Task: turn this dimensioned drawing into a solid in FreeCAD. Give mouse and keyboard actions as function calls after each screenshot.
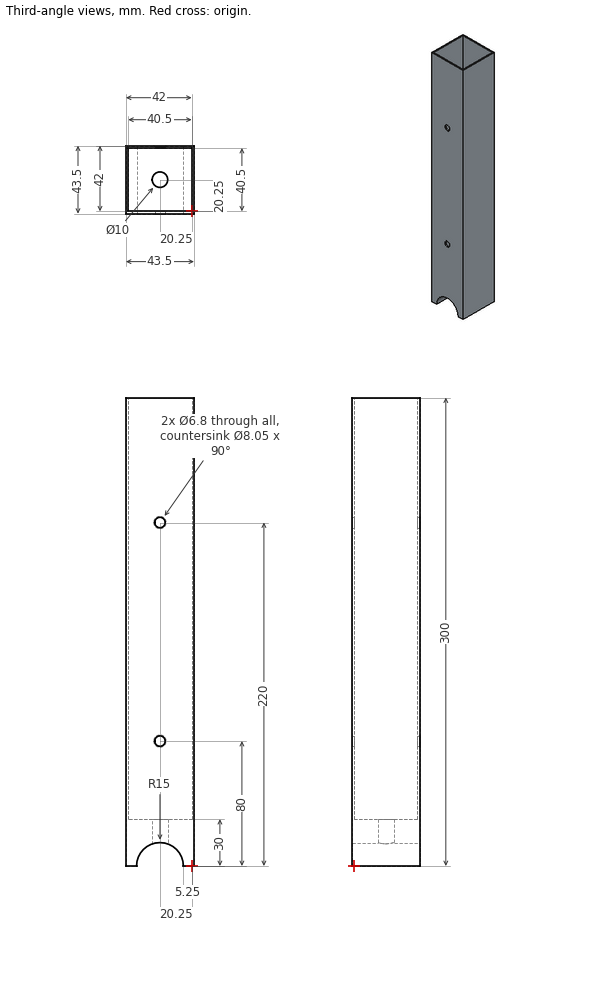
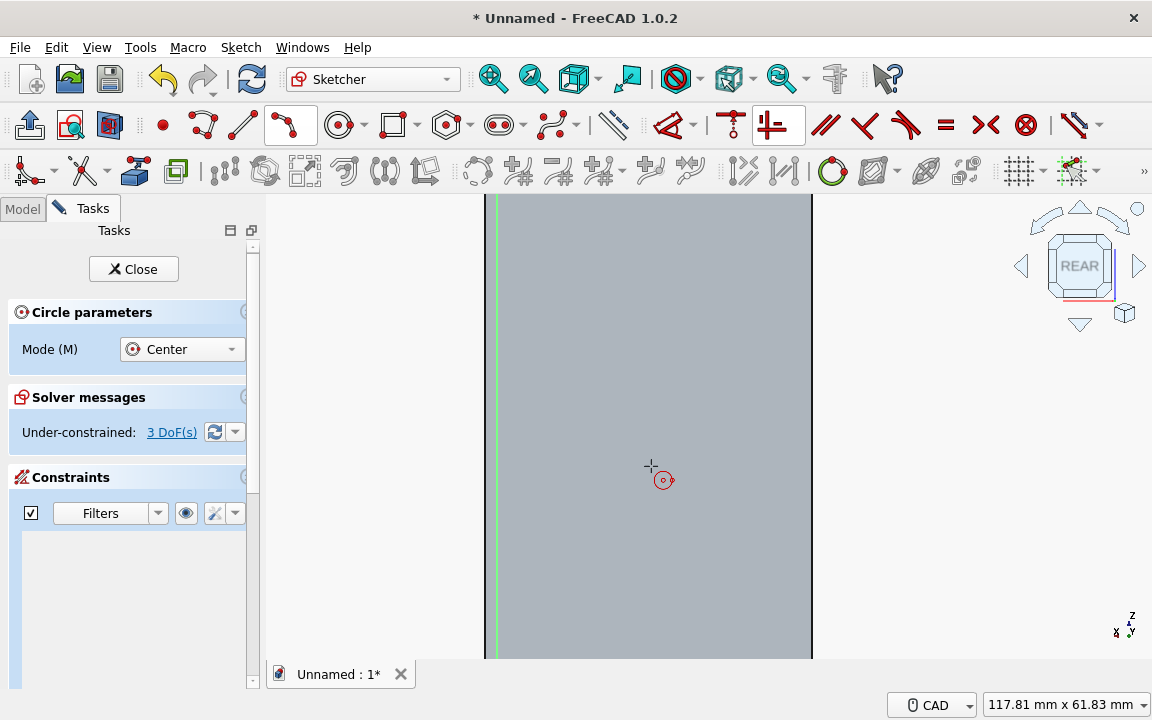
scroll(651, 466, down, 9)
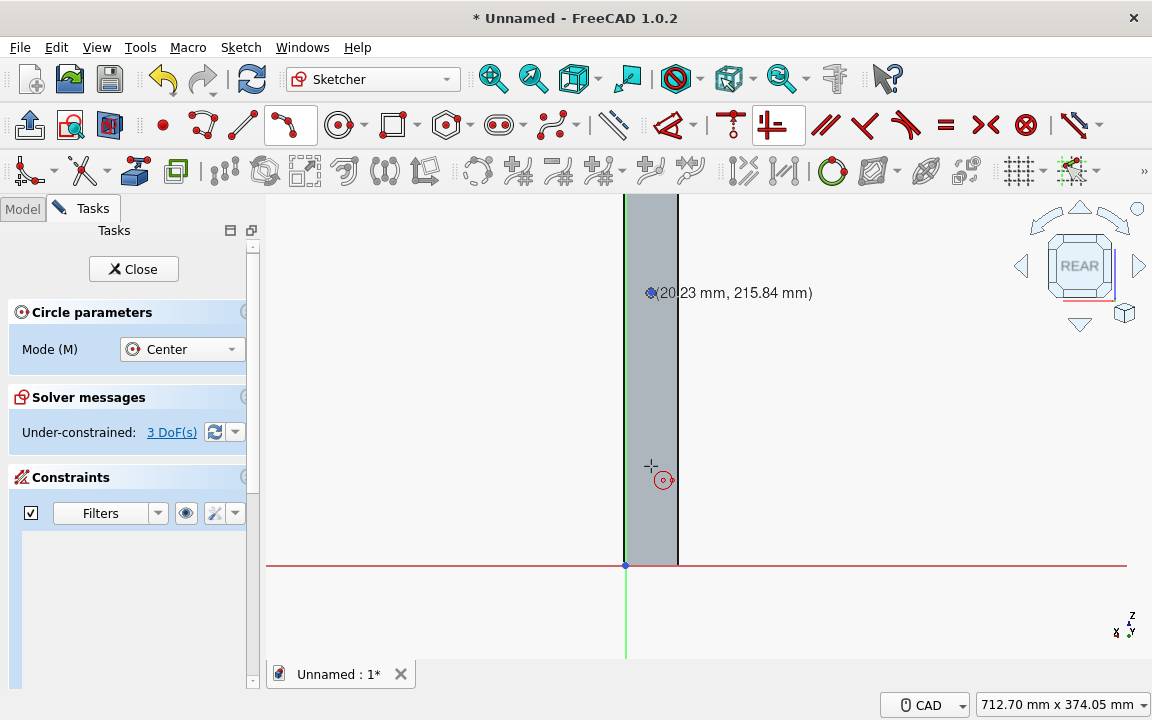
click(651, 466)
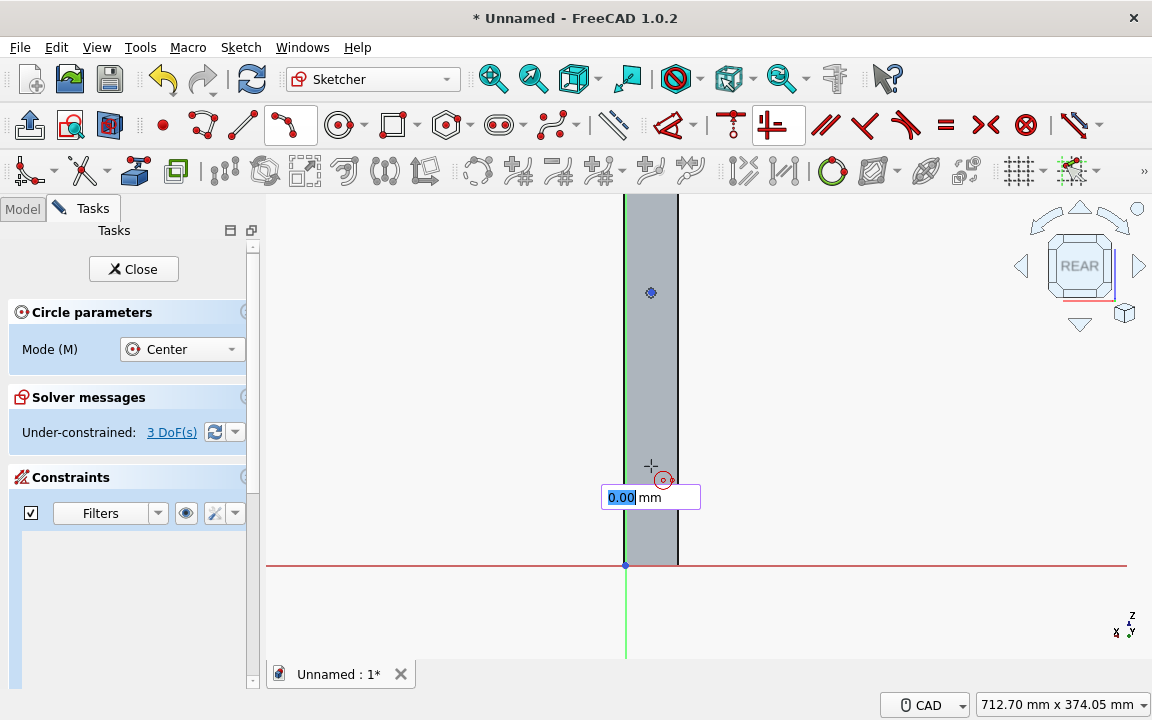
scroll(654, 463, up, 7)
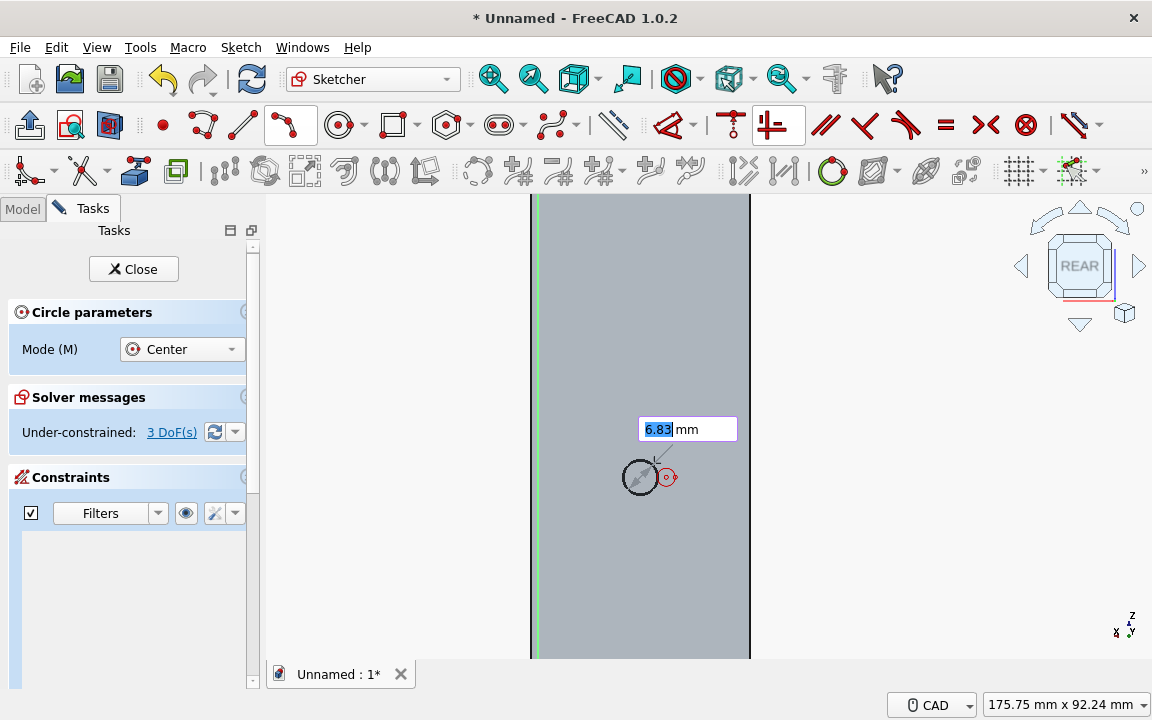
click(653, 463)
key(Escape)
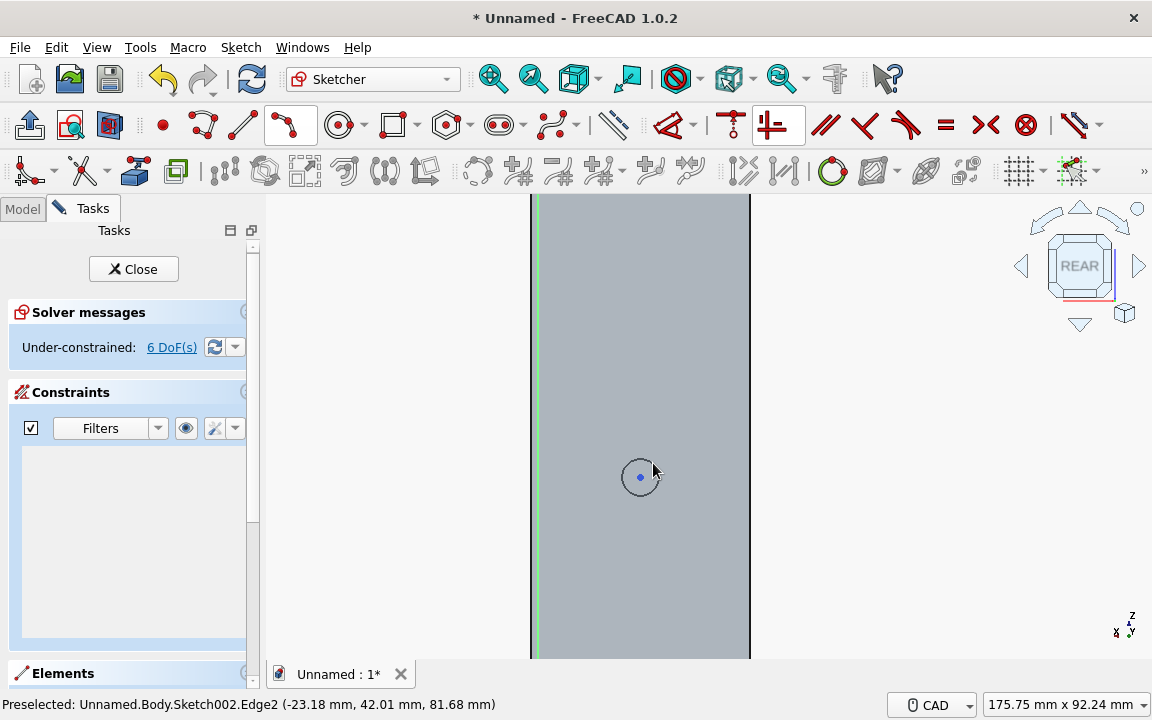
scroll(654, 463, down, 7)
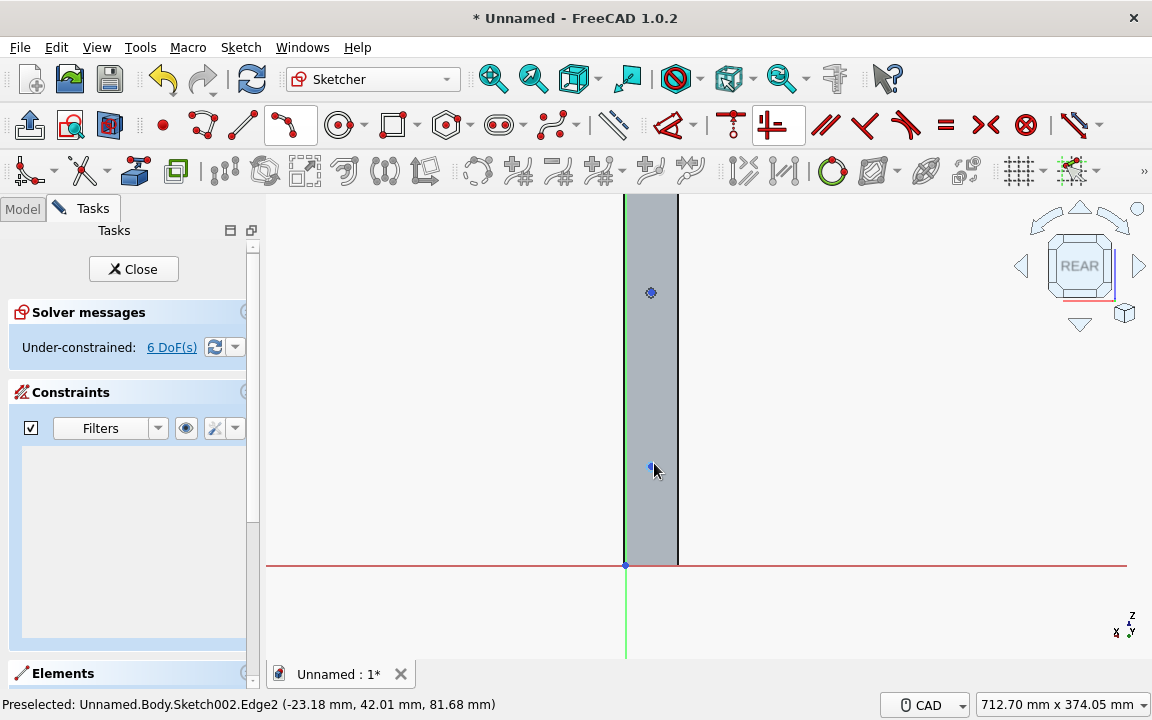
scroll(654, 290, up, 6)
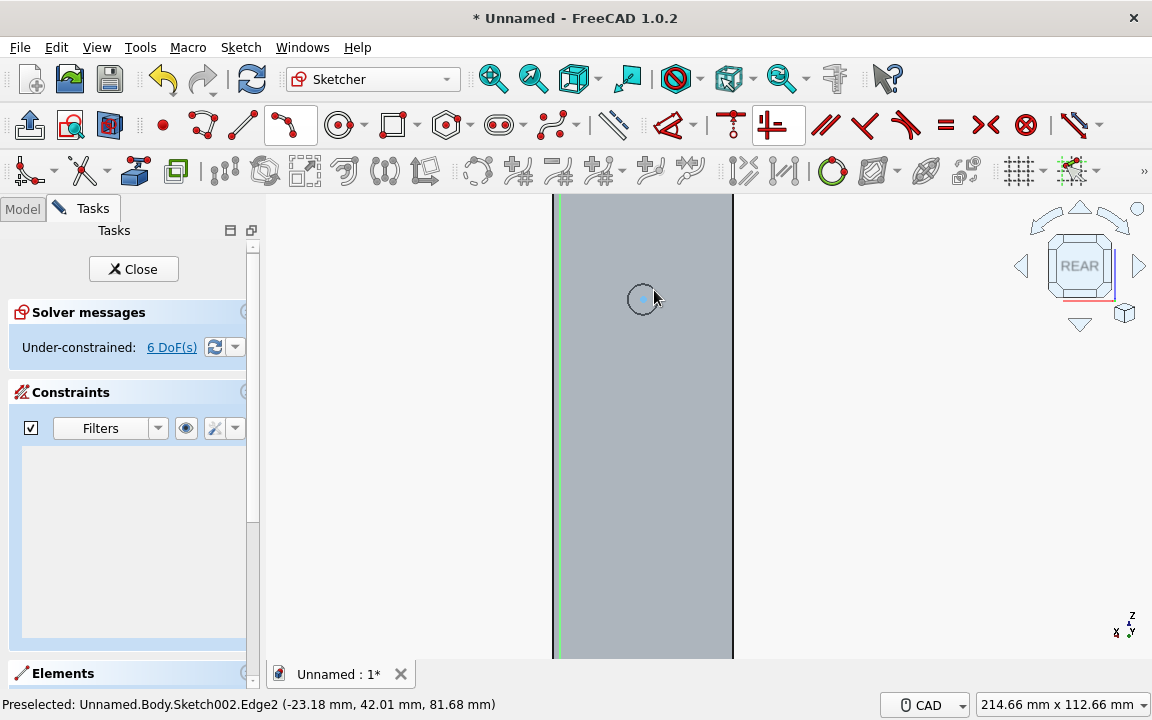
click(654, 289)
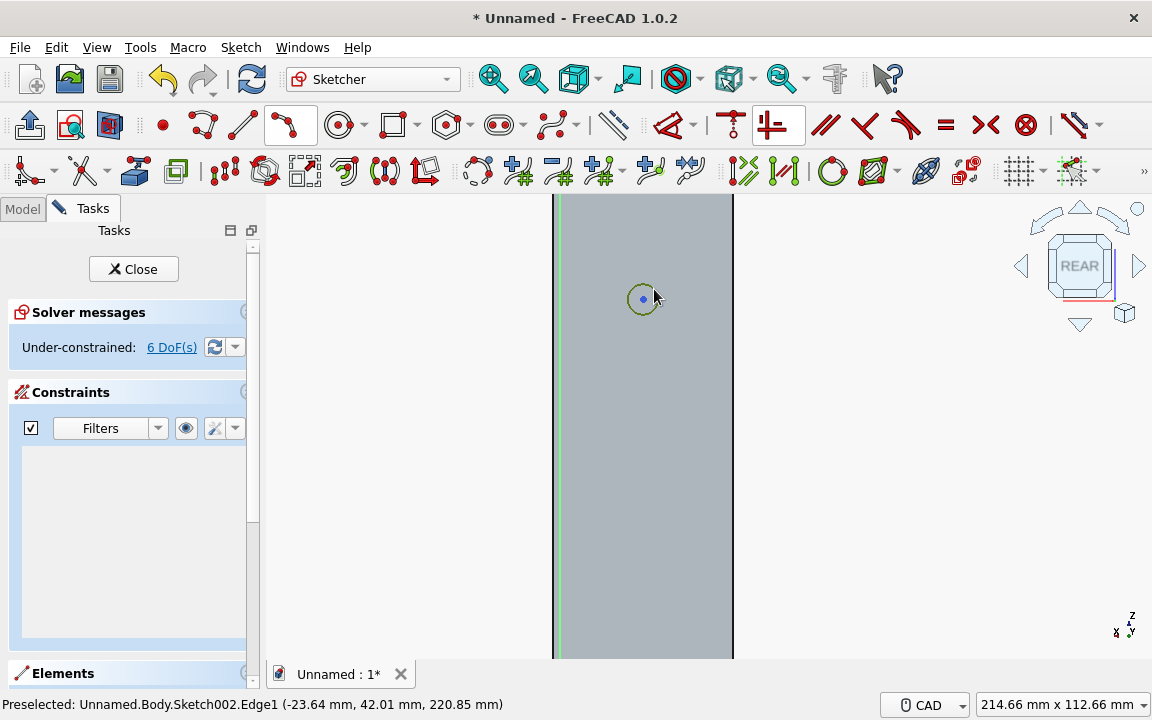
scroll(654, 289, down, 6)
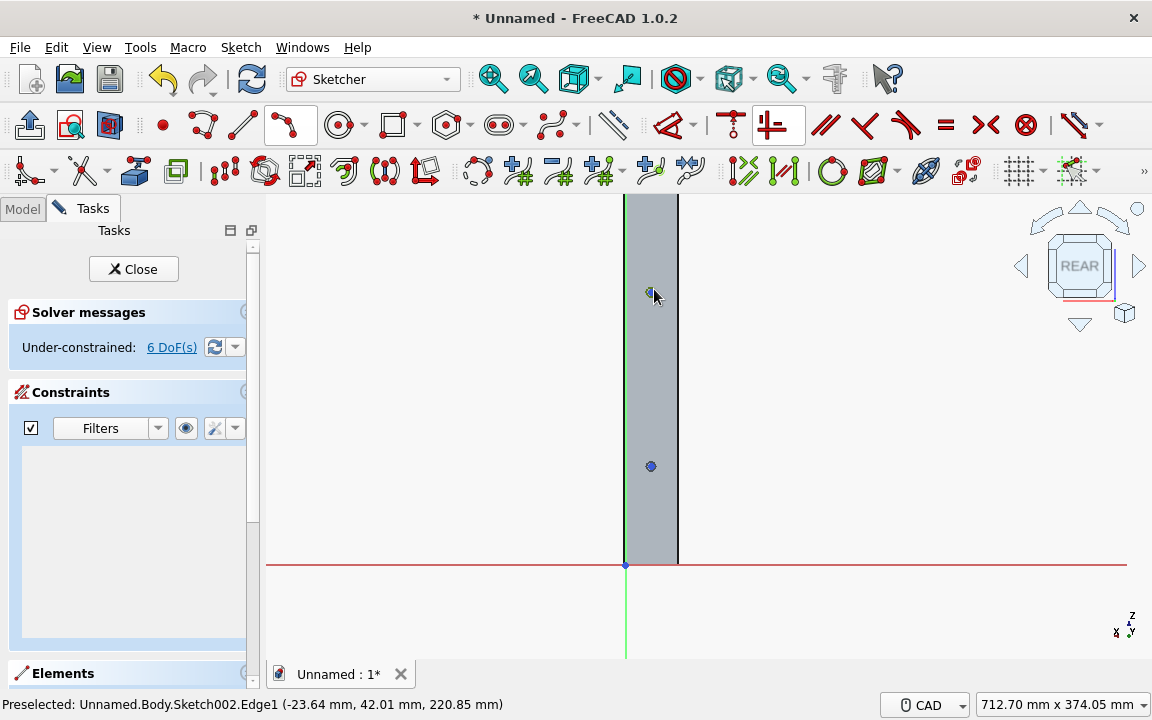
scroll(654, 463, up, 6)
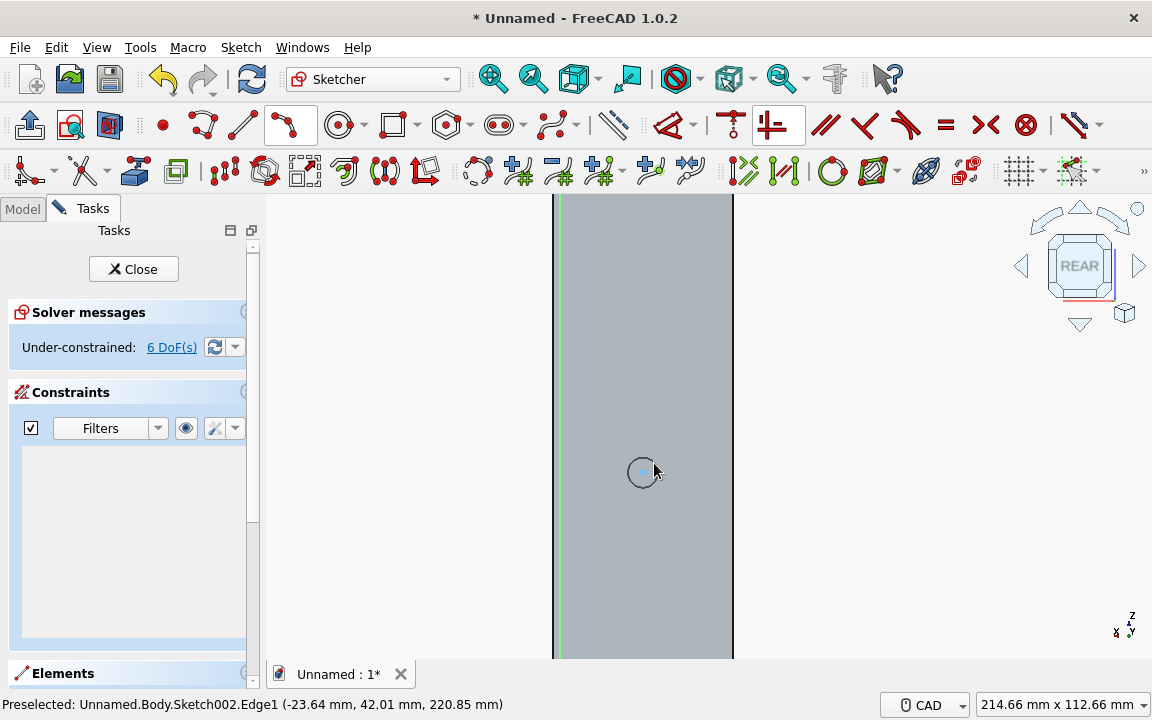
click(654, 462)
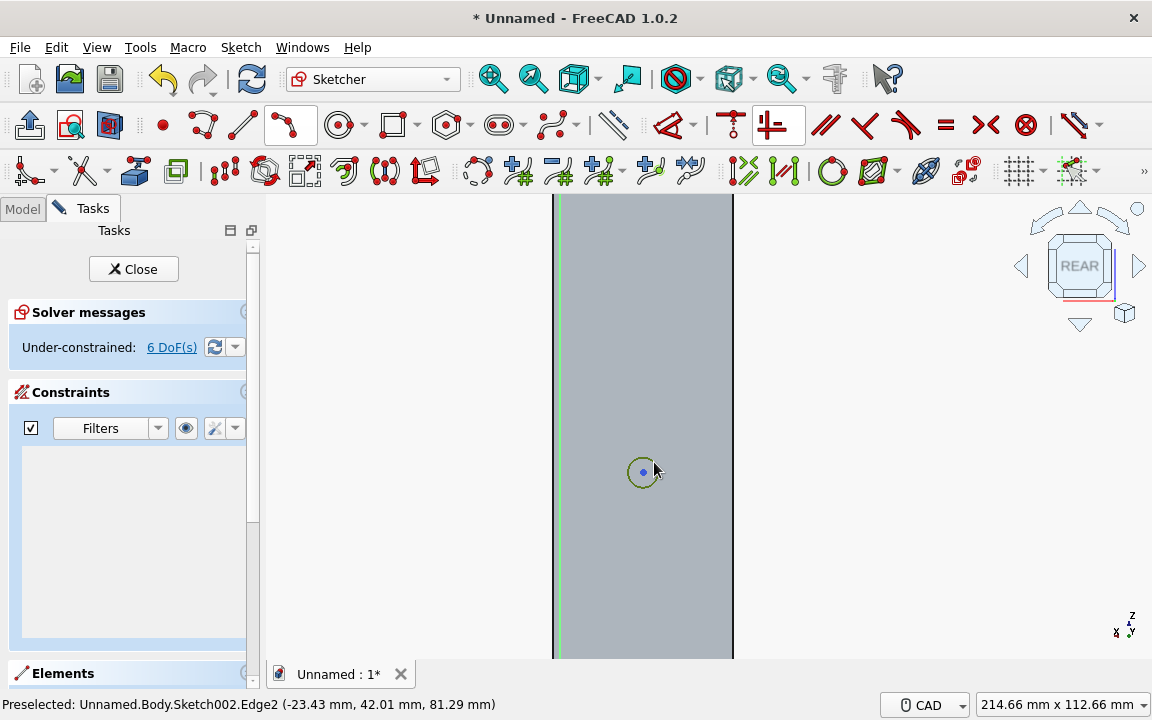
click(946, 126)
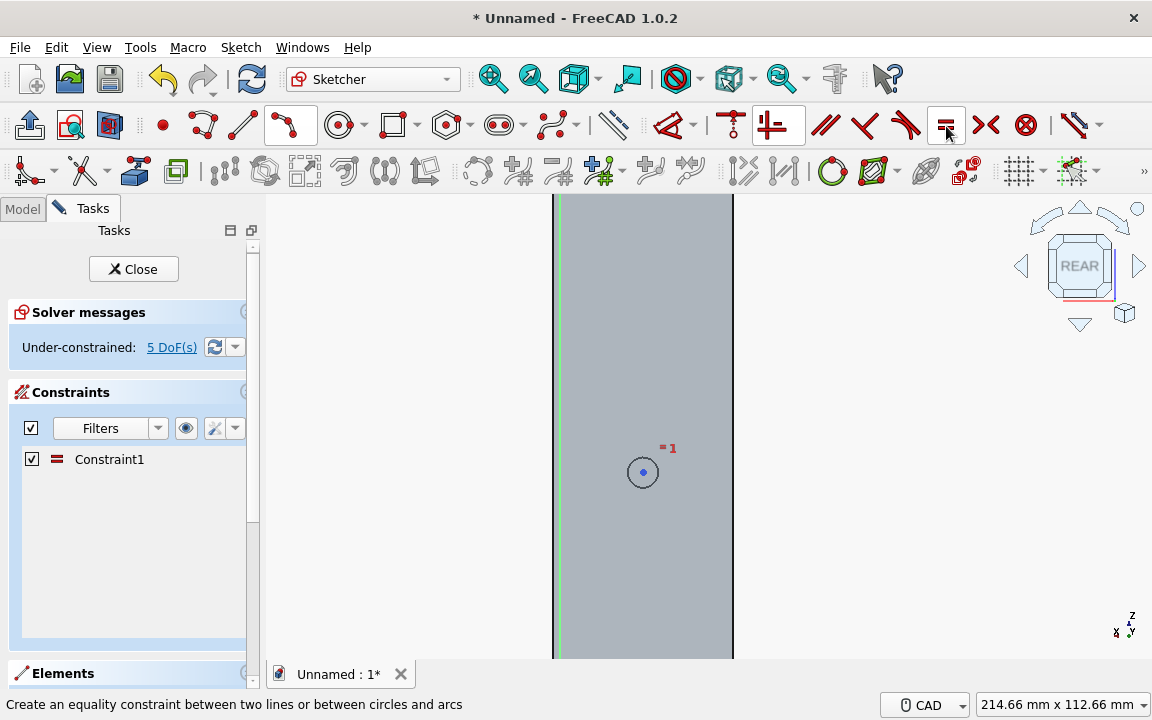
click(668, 126)